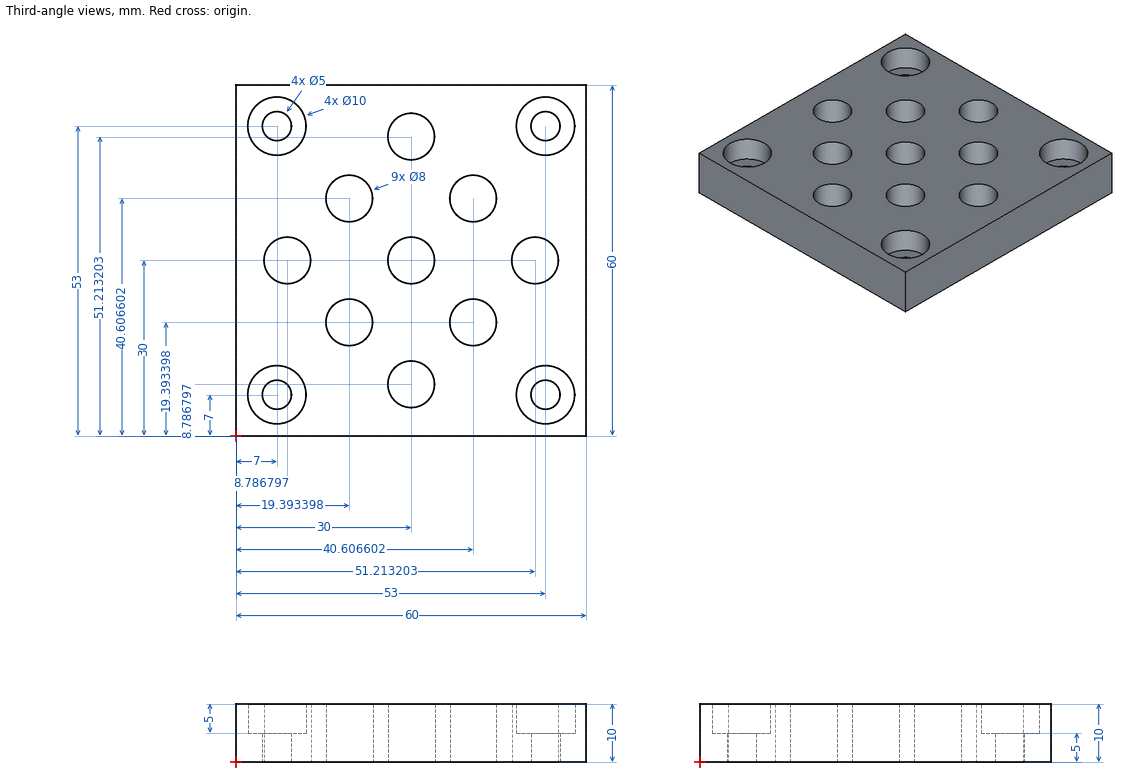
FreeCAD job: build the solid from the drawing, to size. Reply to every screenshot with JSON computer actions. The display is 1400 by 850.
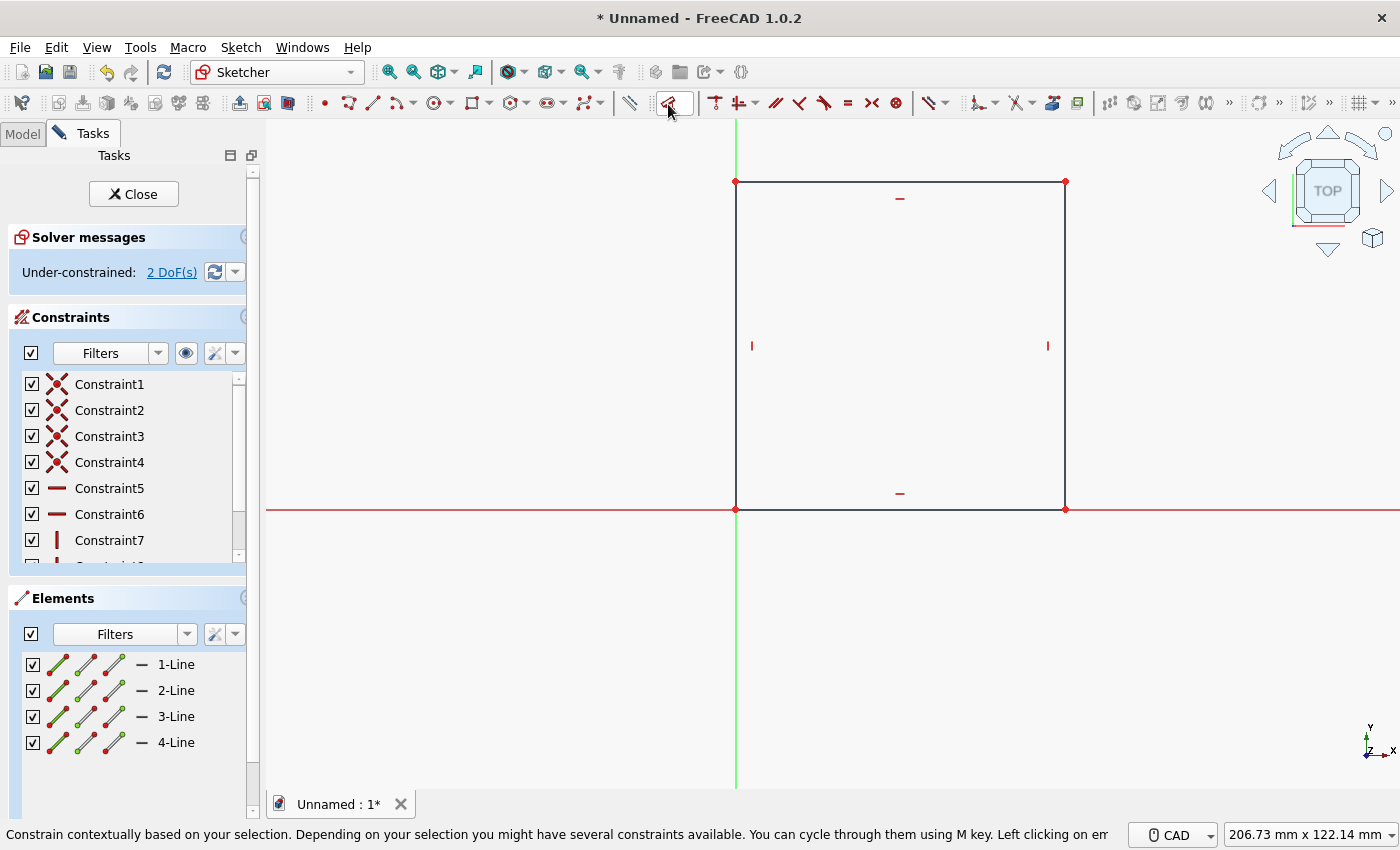
{"action": "left_click", "coordinate": [834, 510]}
{"action": "left_click", "coordinate": [900, 544]}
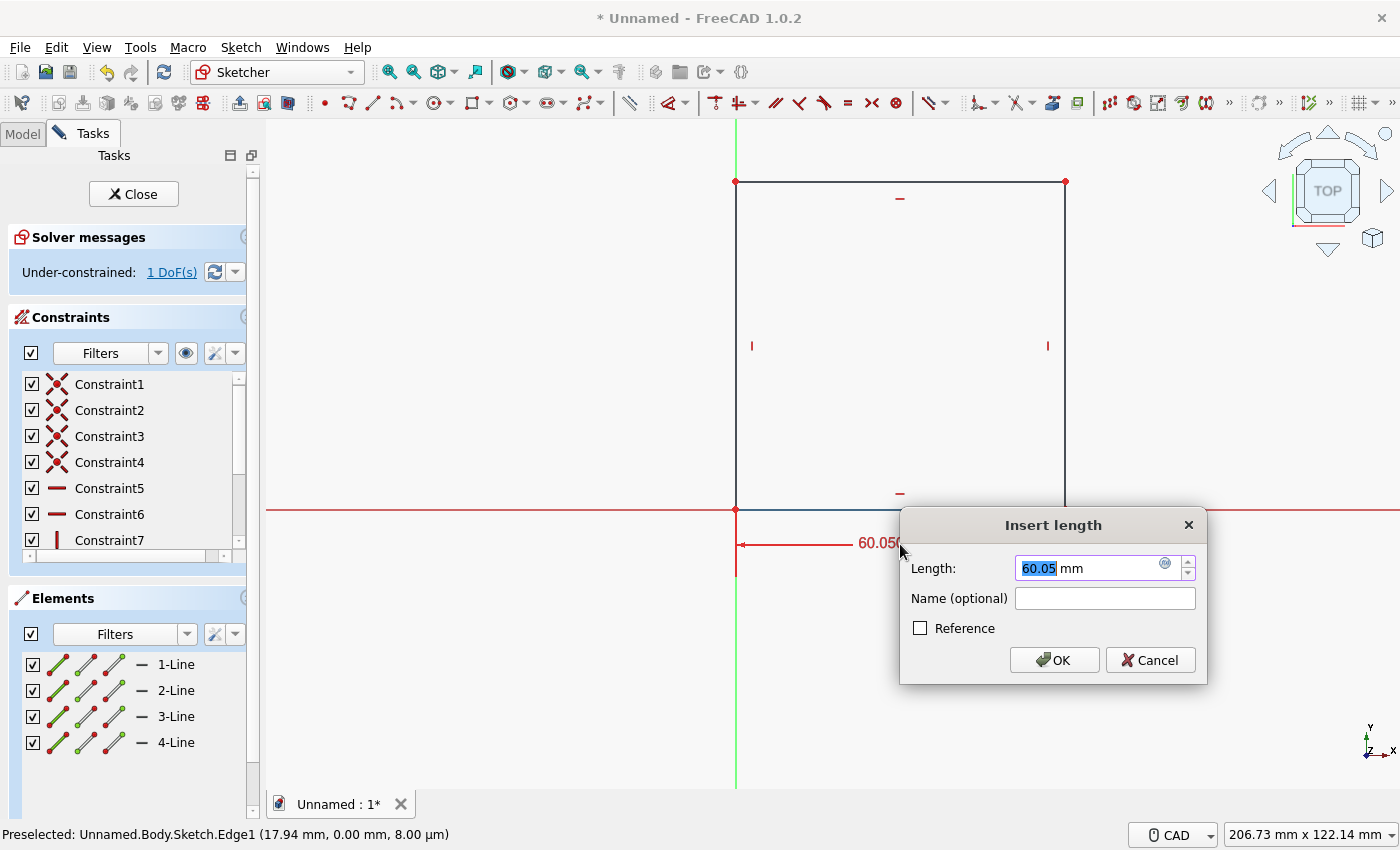
{"action": "type", "text": "60"}
{"action": "key", "text": "Return"}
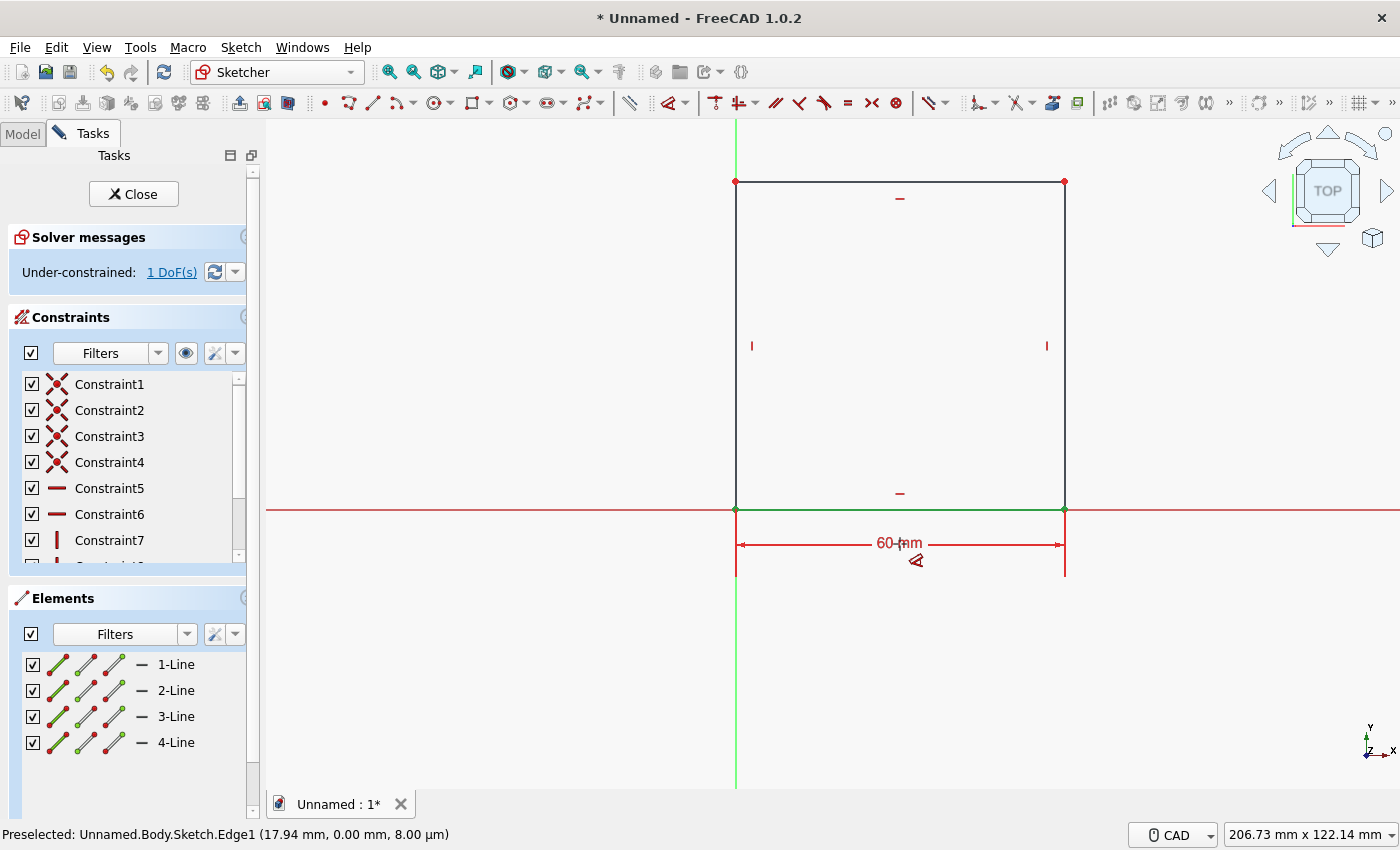
{"action": "left_click", "coordinate": [1065, 411]}
{"action": "left_click", "coordinate": [1099, 346]}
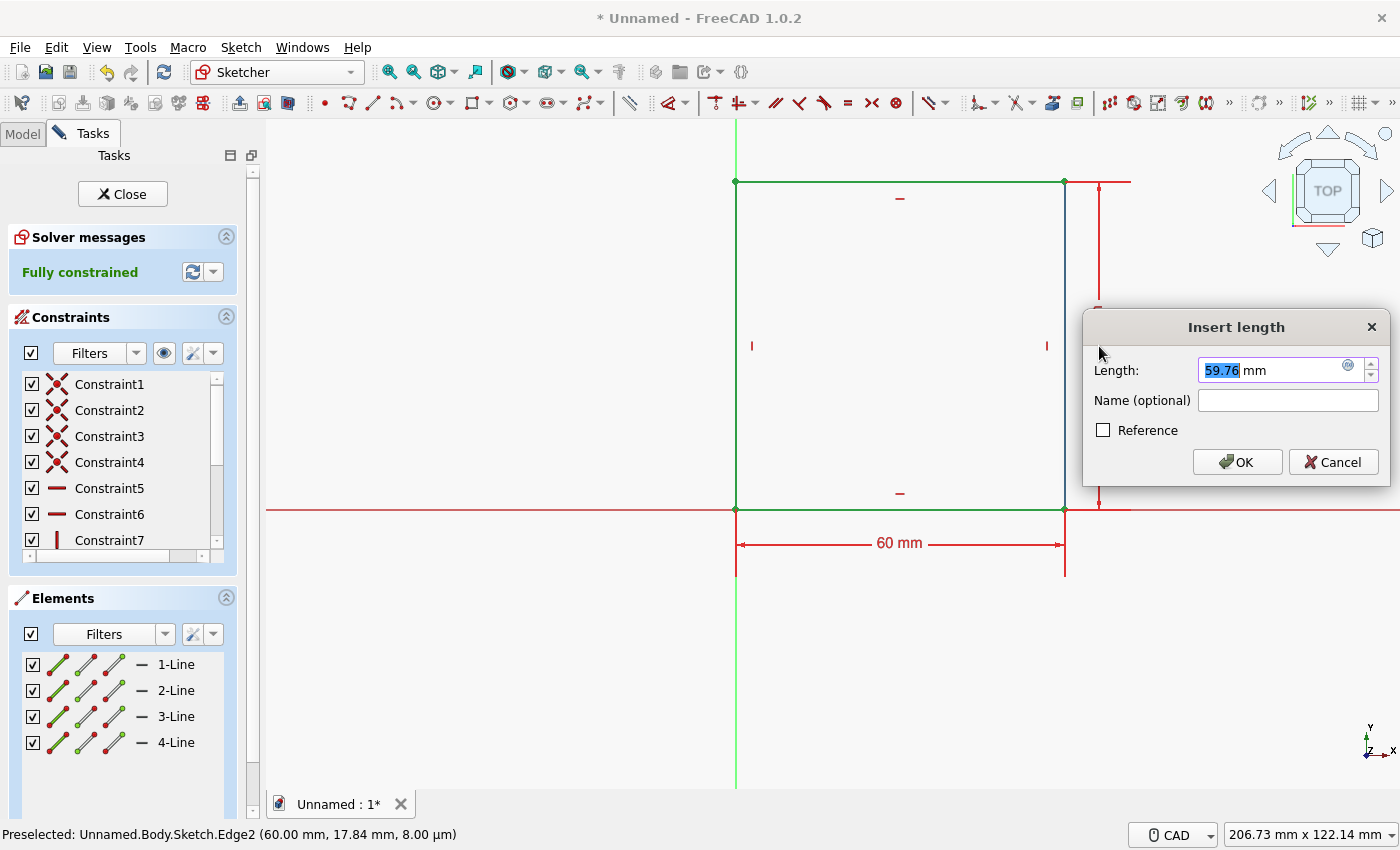
{"action": "type", "text": "60"}
{"action": "key", "text": "Return"}
{"action": "key", "text": "Escape"}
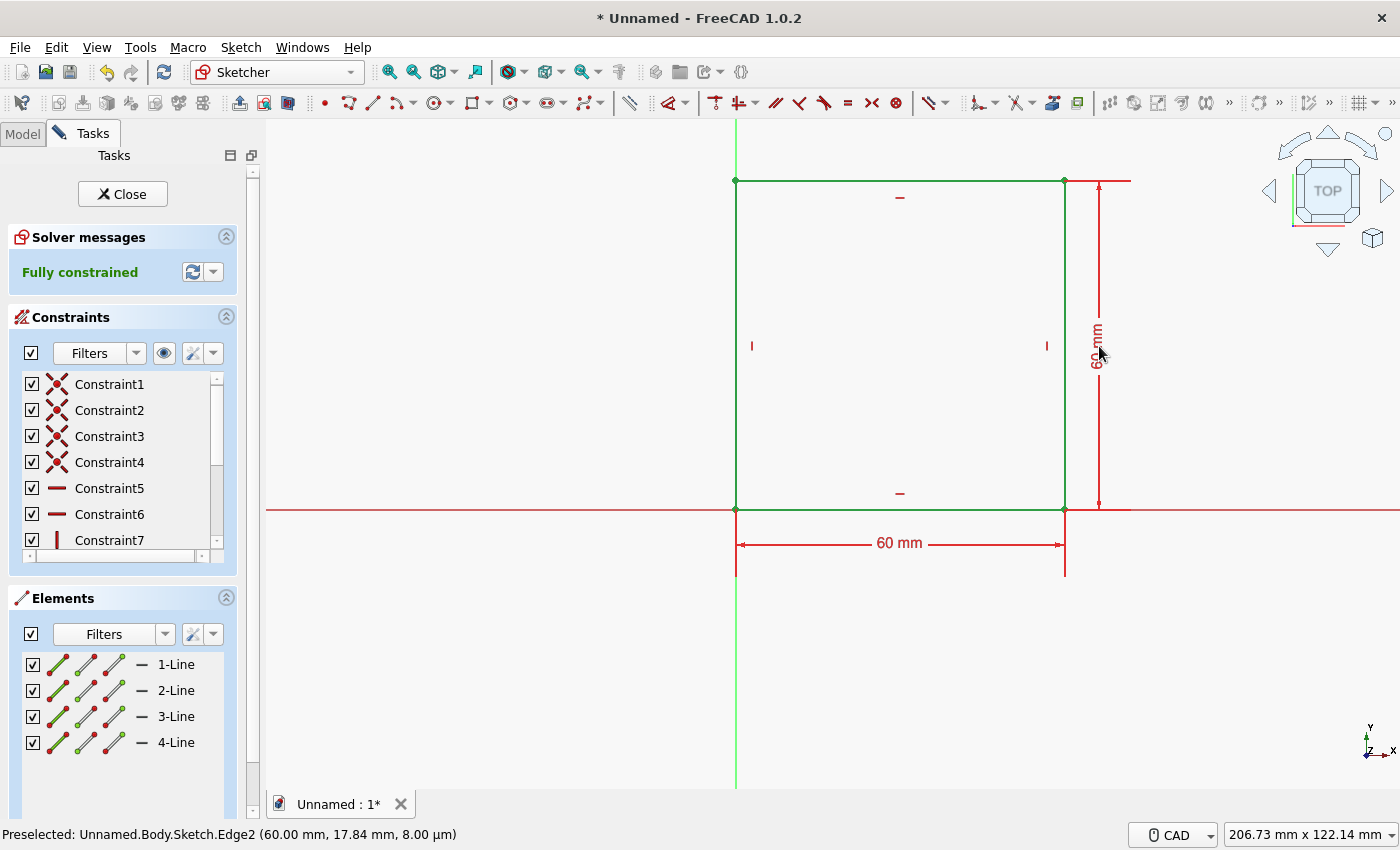
{"action": "left_click", "coordinate": [123, 194]}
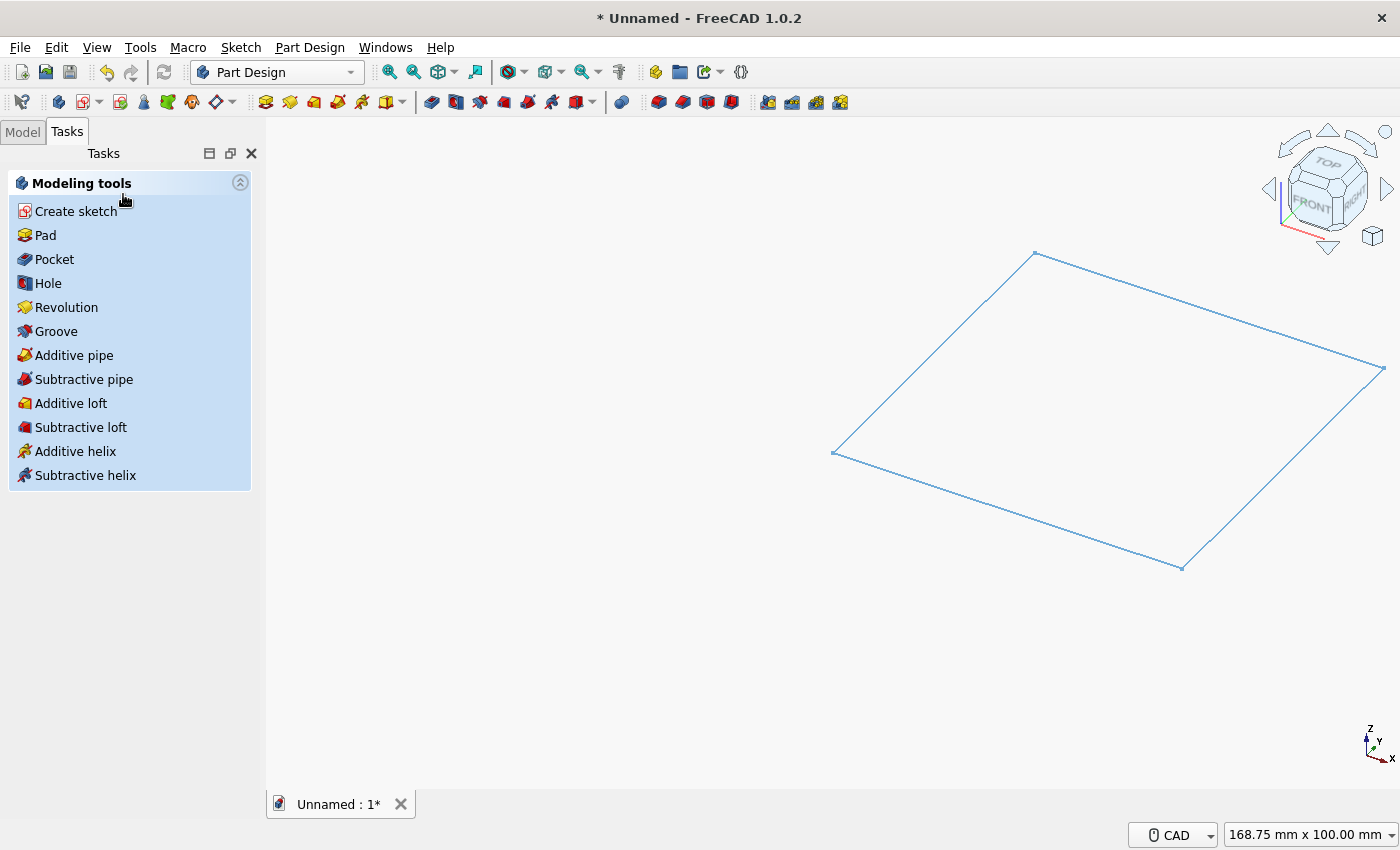
{"action": "left_click", "coordinate": [266, 102]}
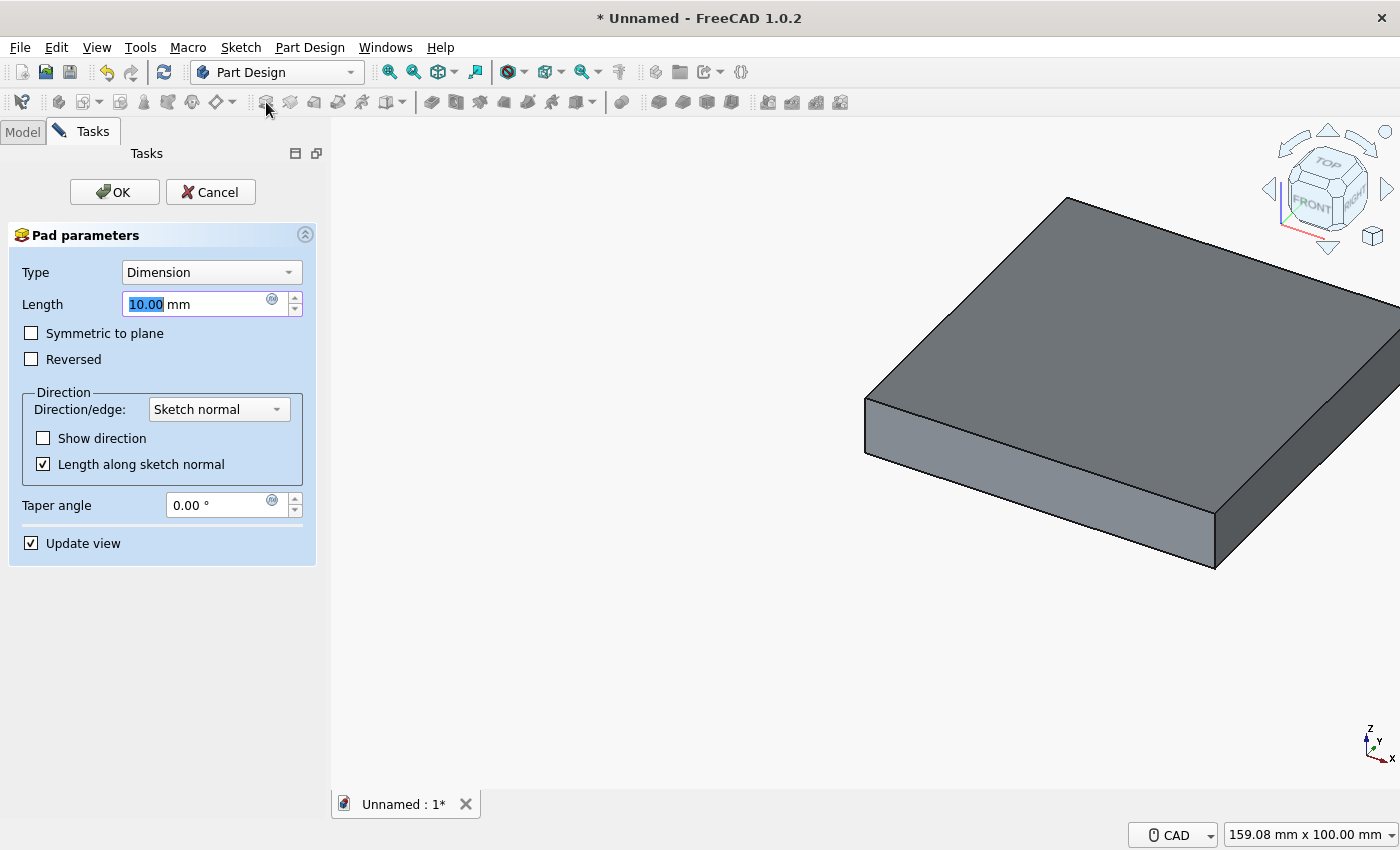
{"action": "type", "text": "10"}
{"action": "key", "text": "Tab"}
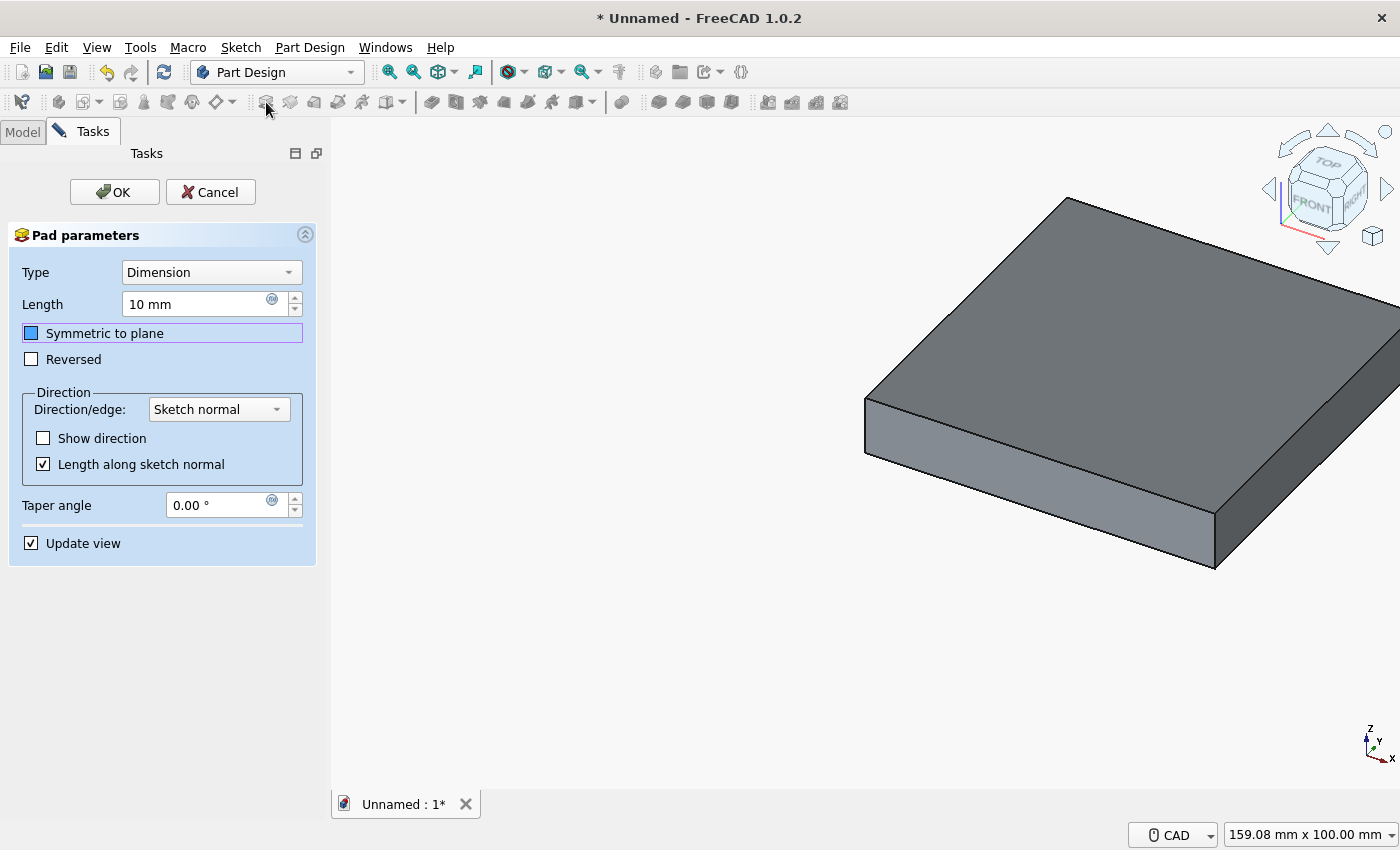
{"action": "left_click", "coordinate": [115, 192]}